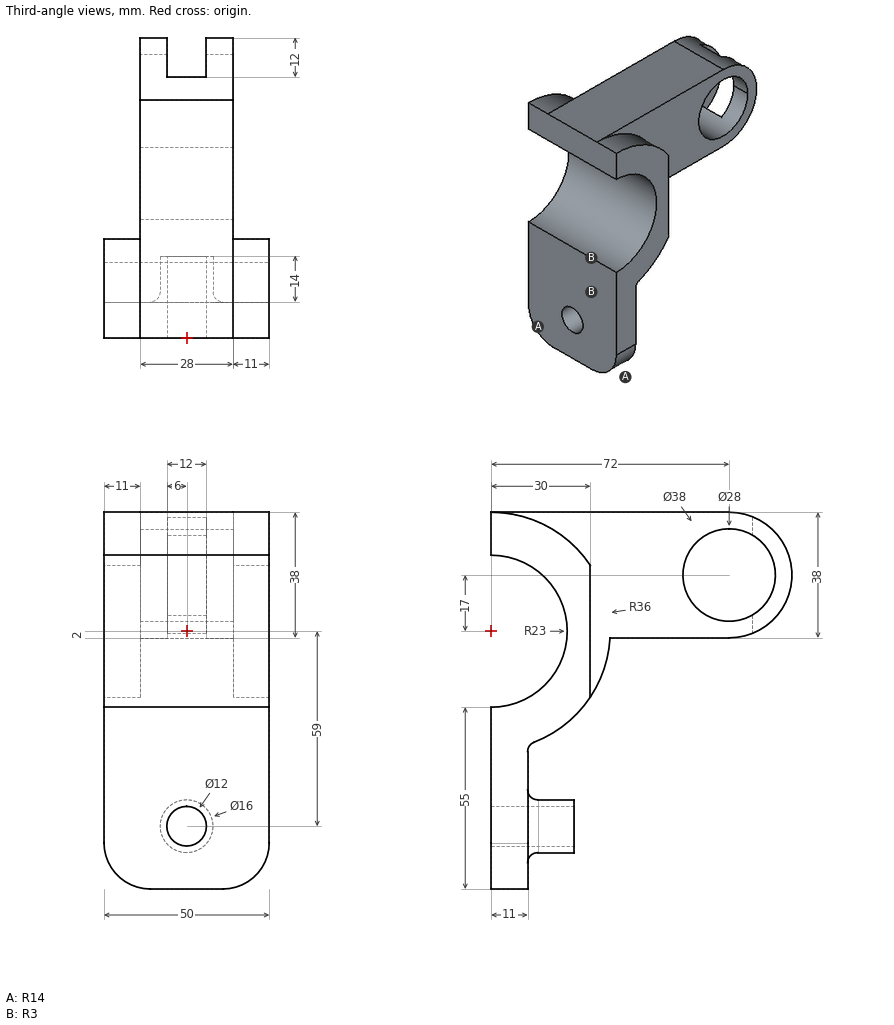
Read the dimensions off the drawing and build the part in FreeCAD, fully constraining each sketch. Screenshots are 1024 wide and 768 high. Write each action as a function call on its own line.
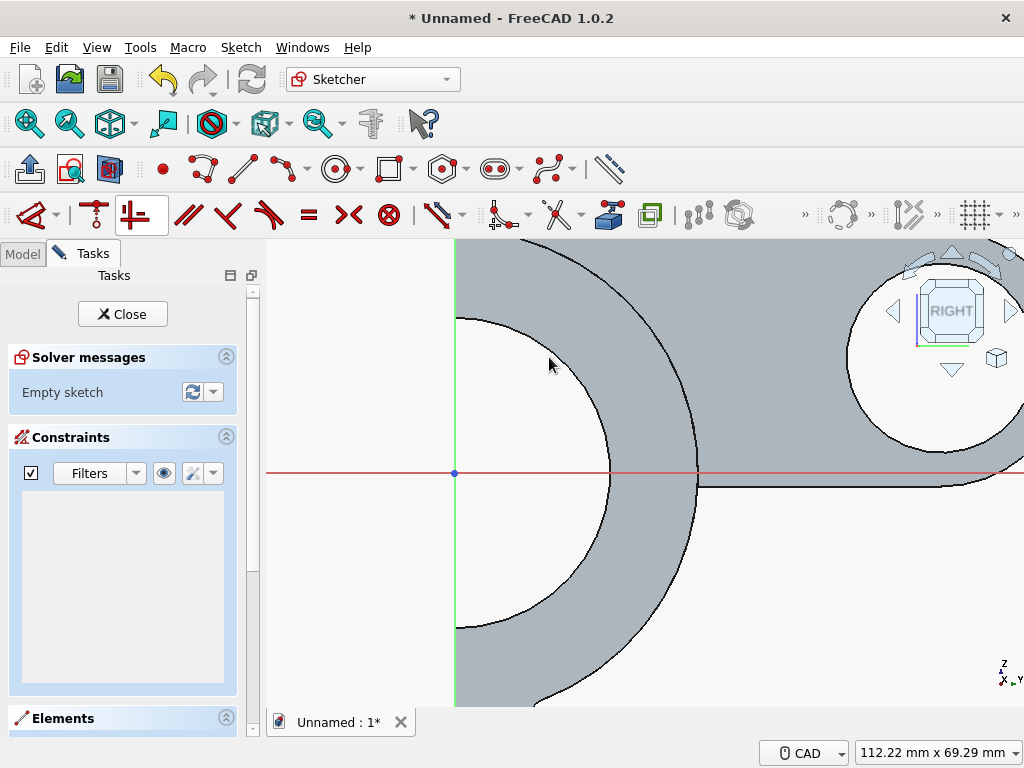
click(244, 170)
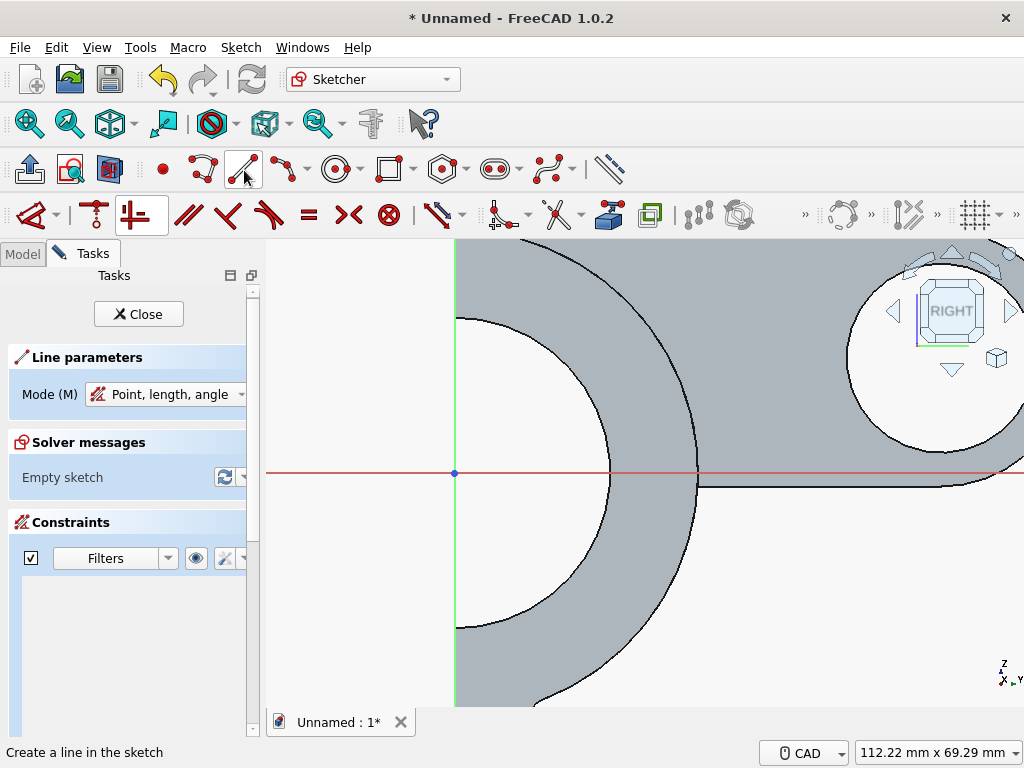
click(657, 339)
click(657, 607)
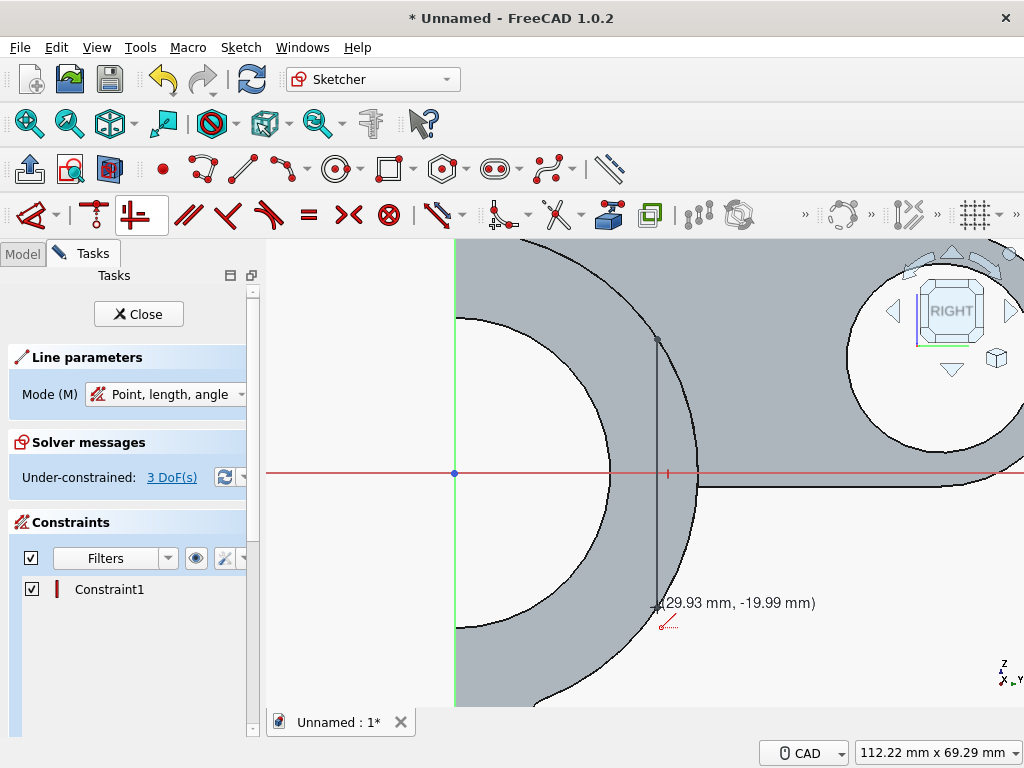
click(284, 170)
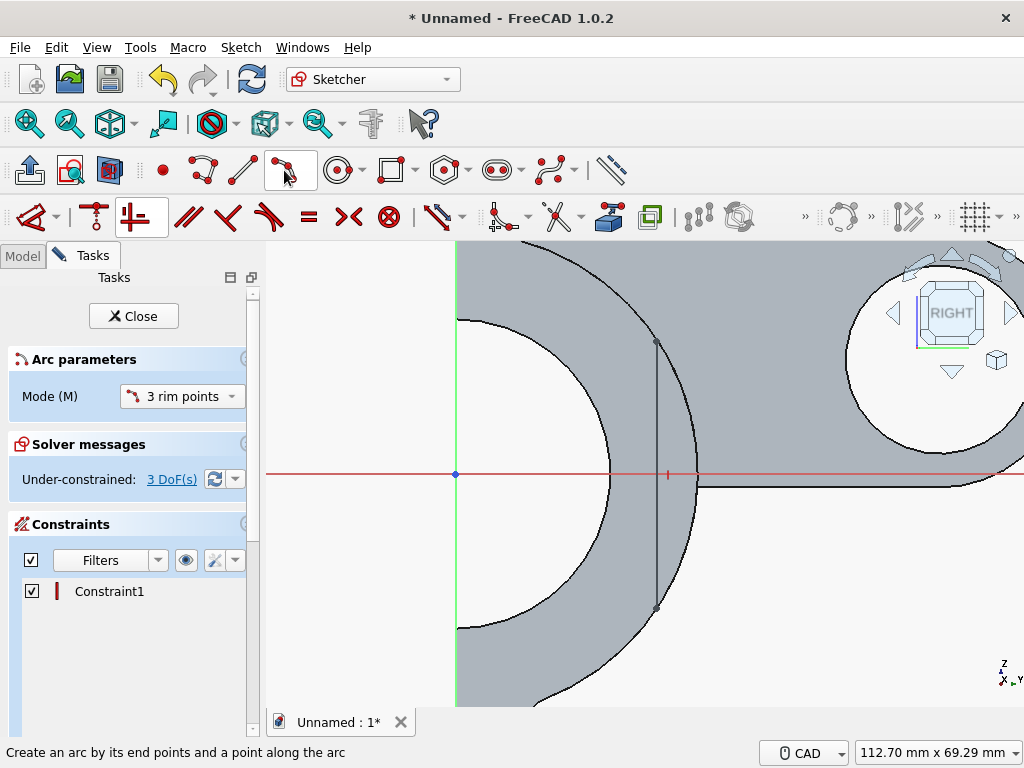
click(657, 608)
click(657, 342)
click(696, 502)
key(Escape)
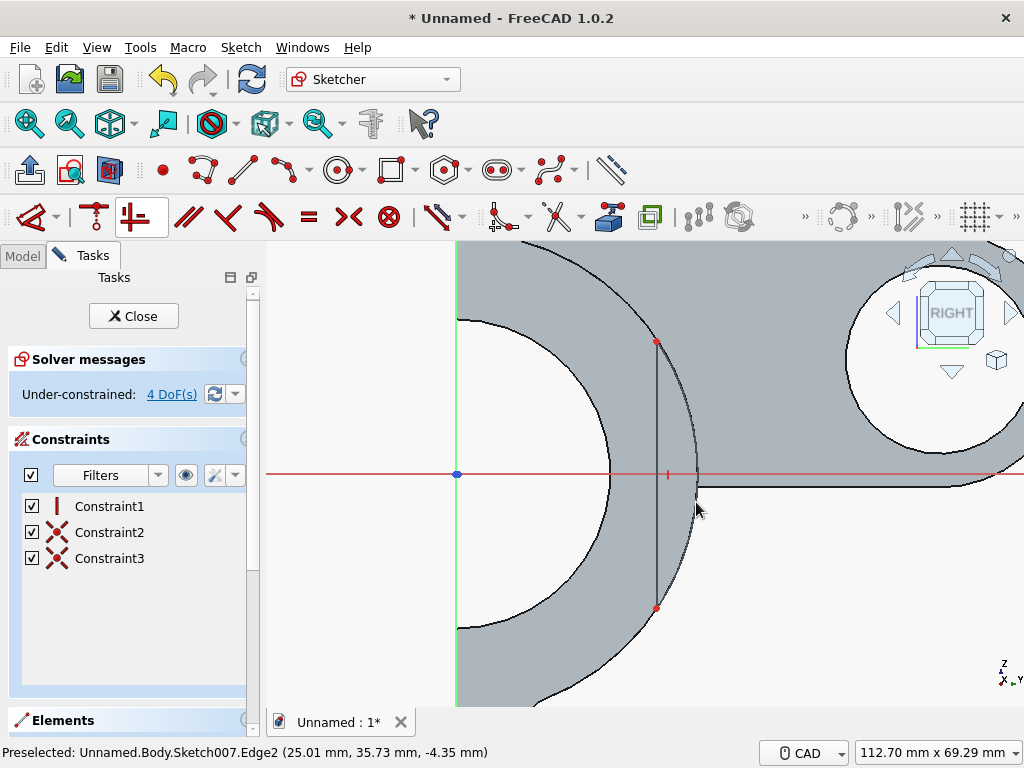
drag(446, 464, 469, 485)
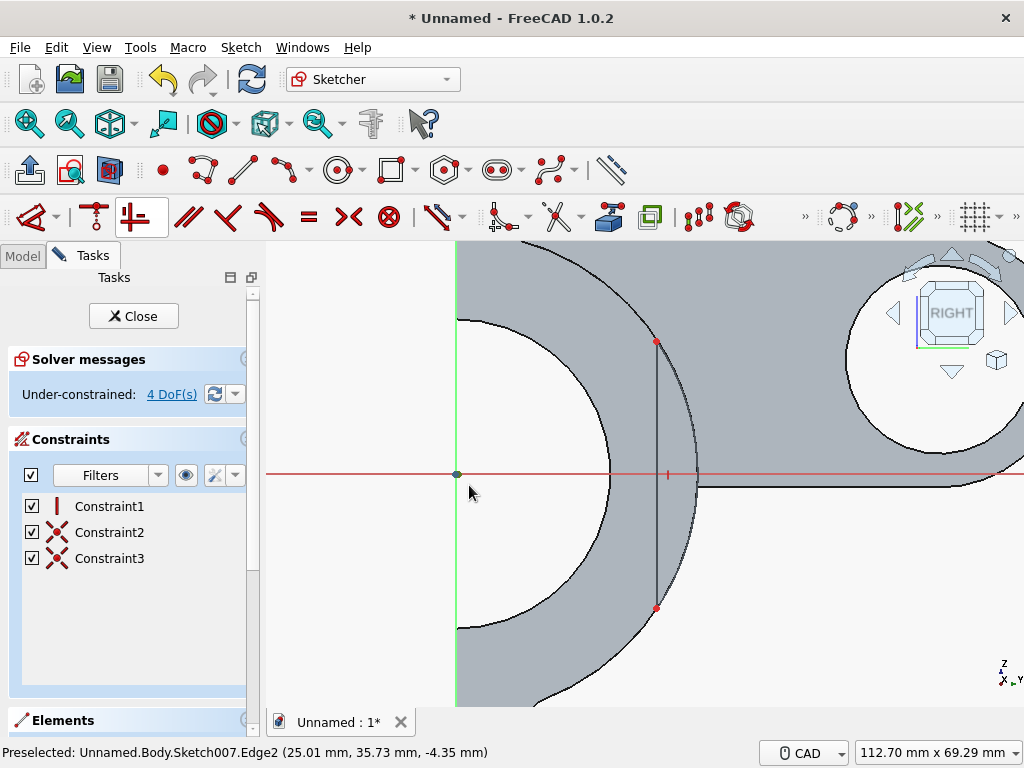
click(94, 218)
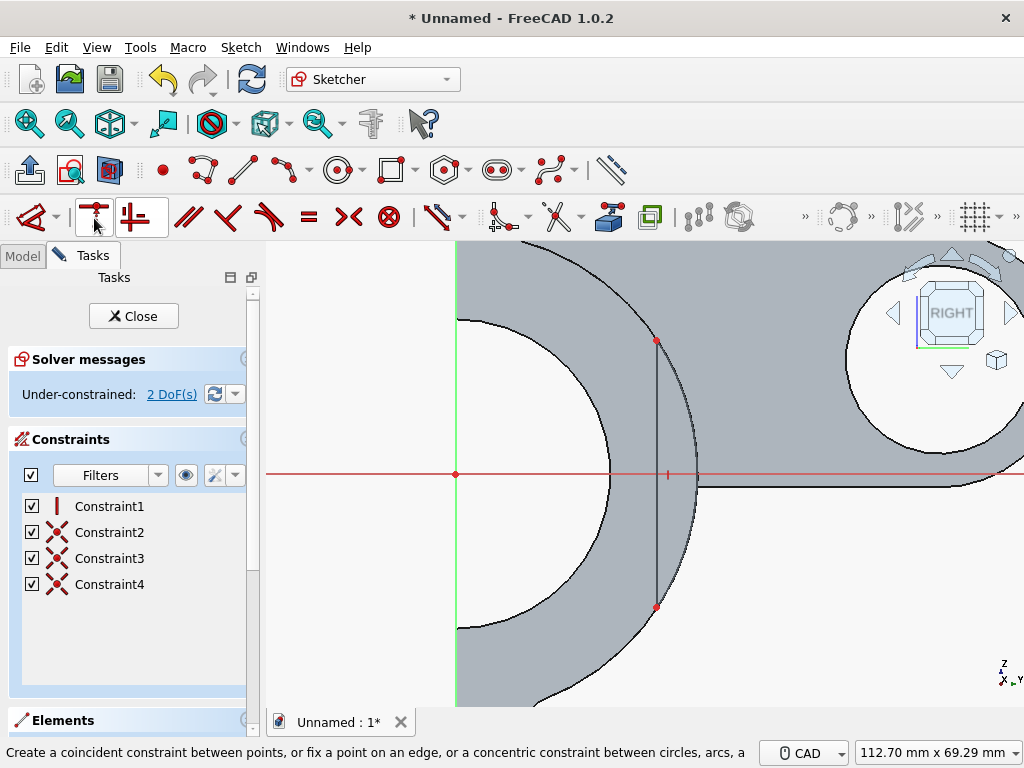
click(32, 218)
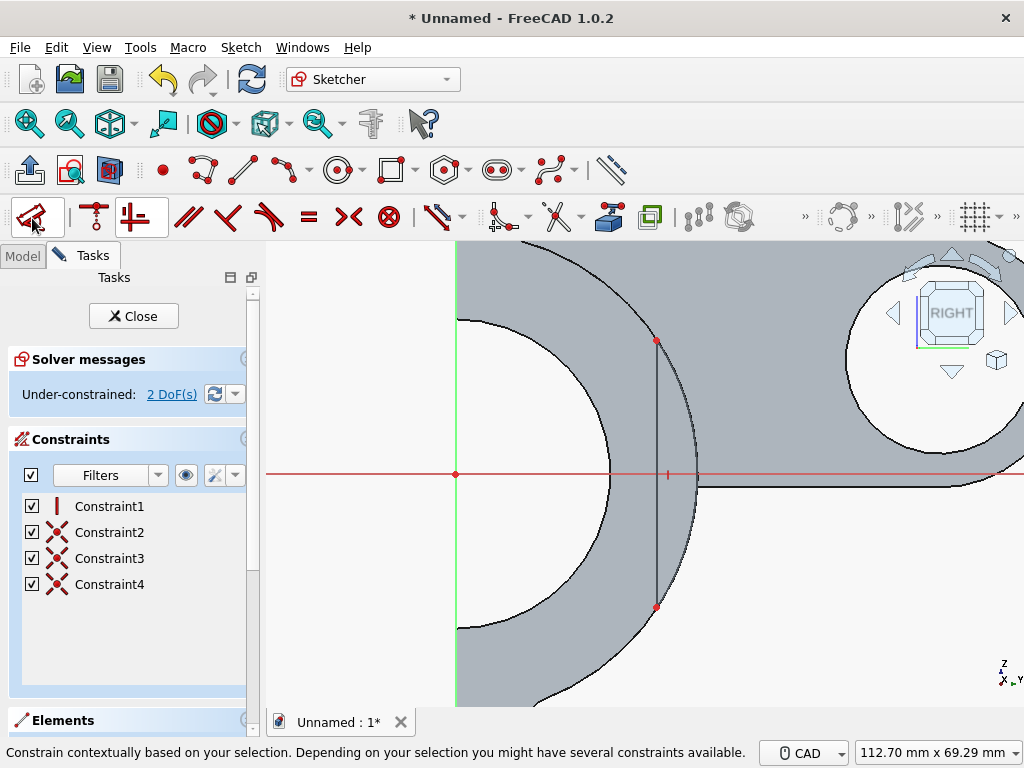
click(691, 530)
click(722, 537)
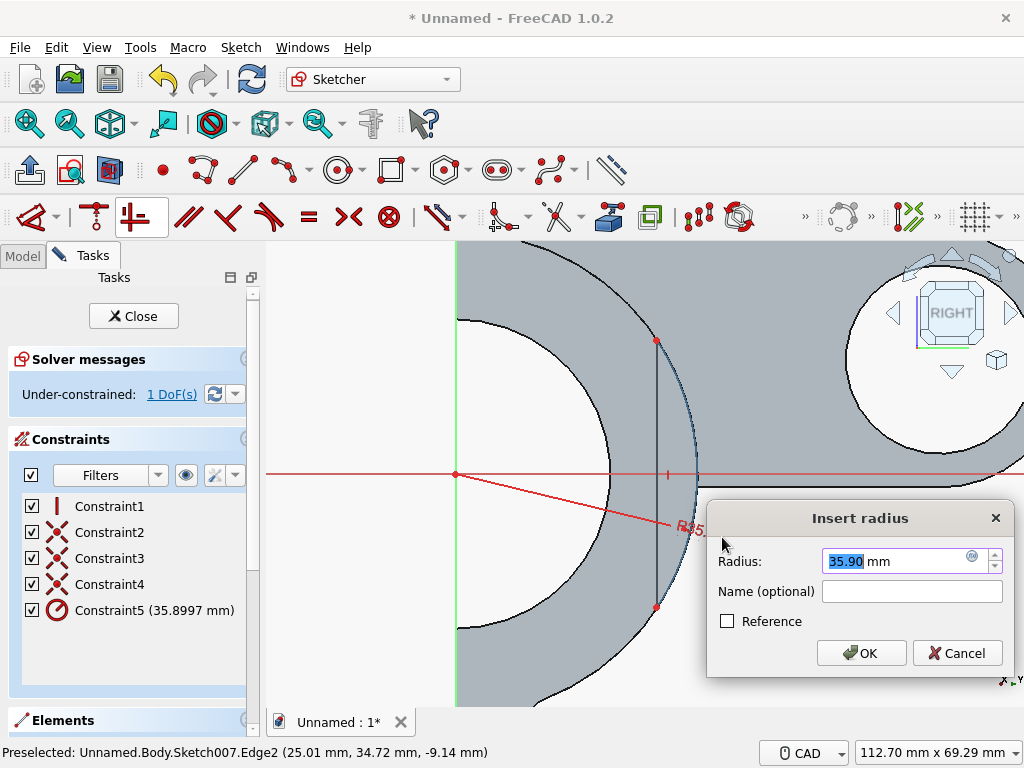
text(36)
key(Return)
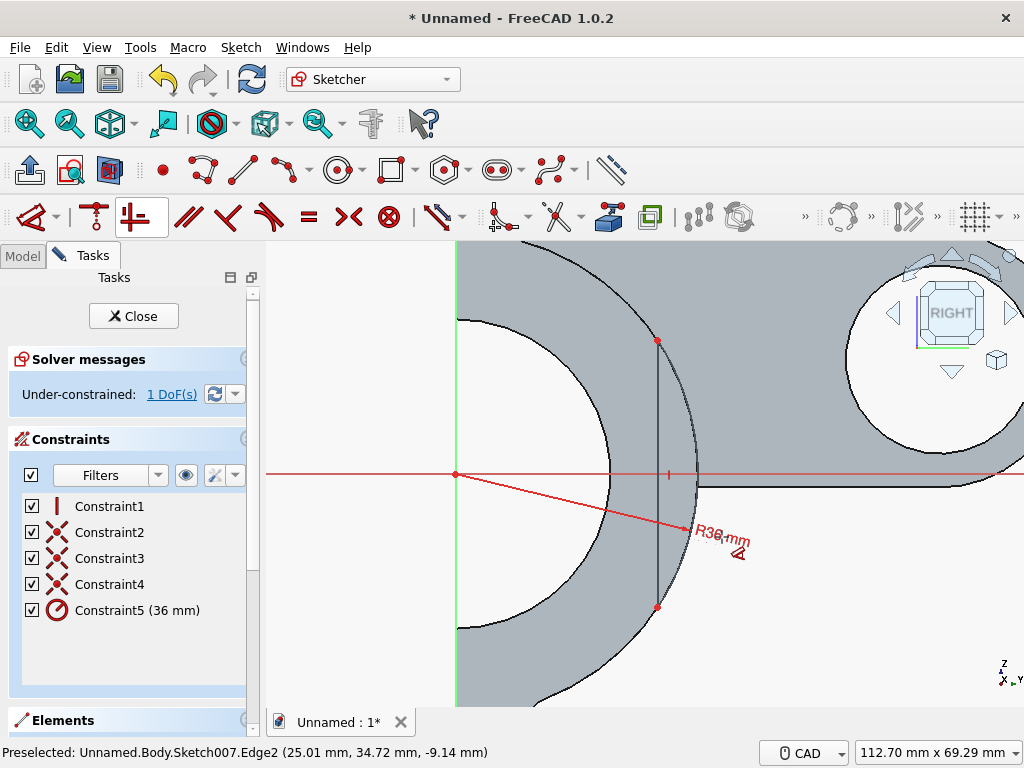
click(658, 341)
click(557, 307)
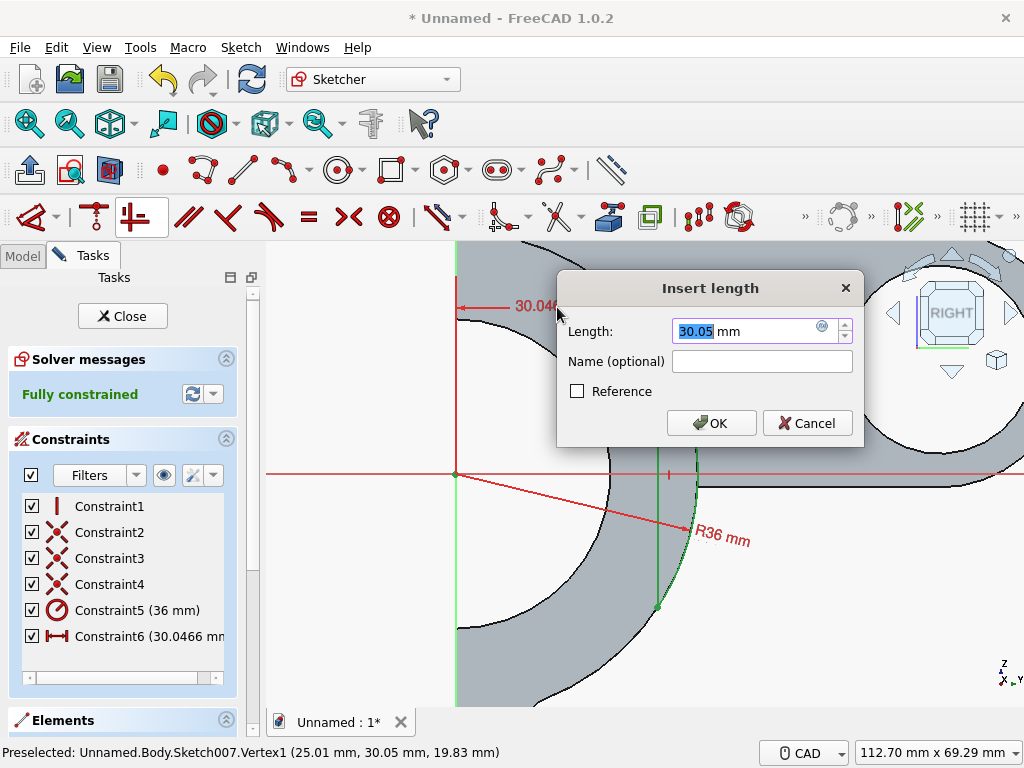
text(30)
key(Return)
key(Escape)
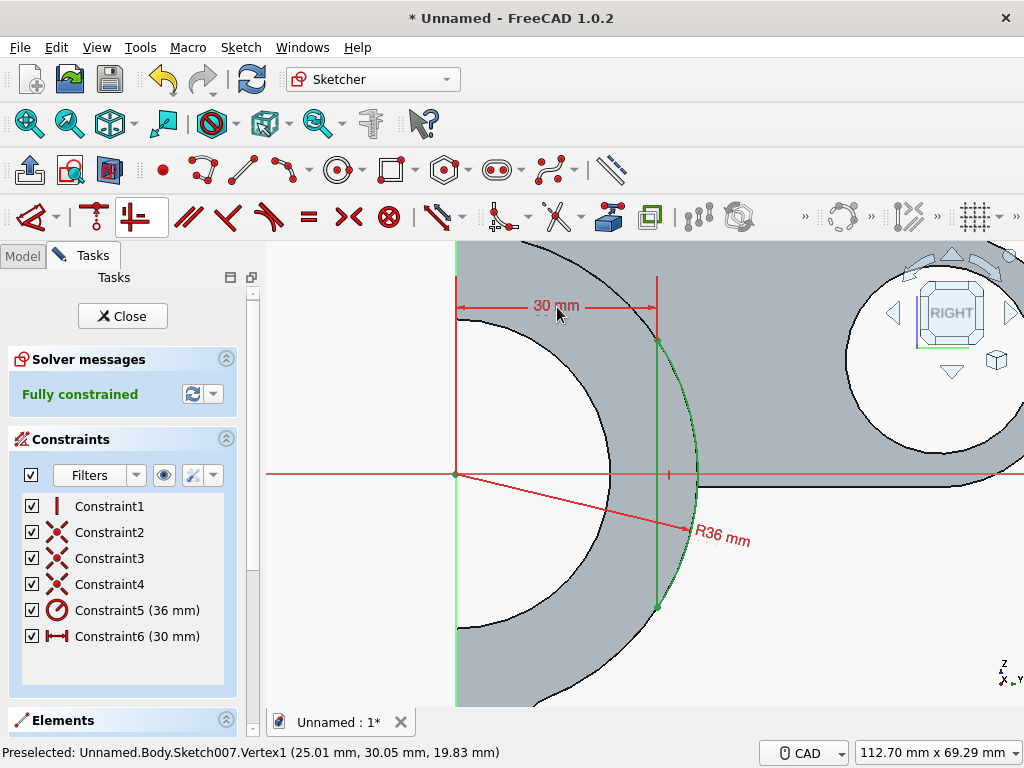
click(123, 316)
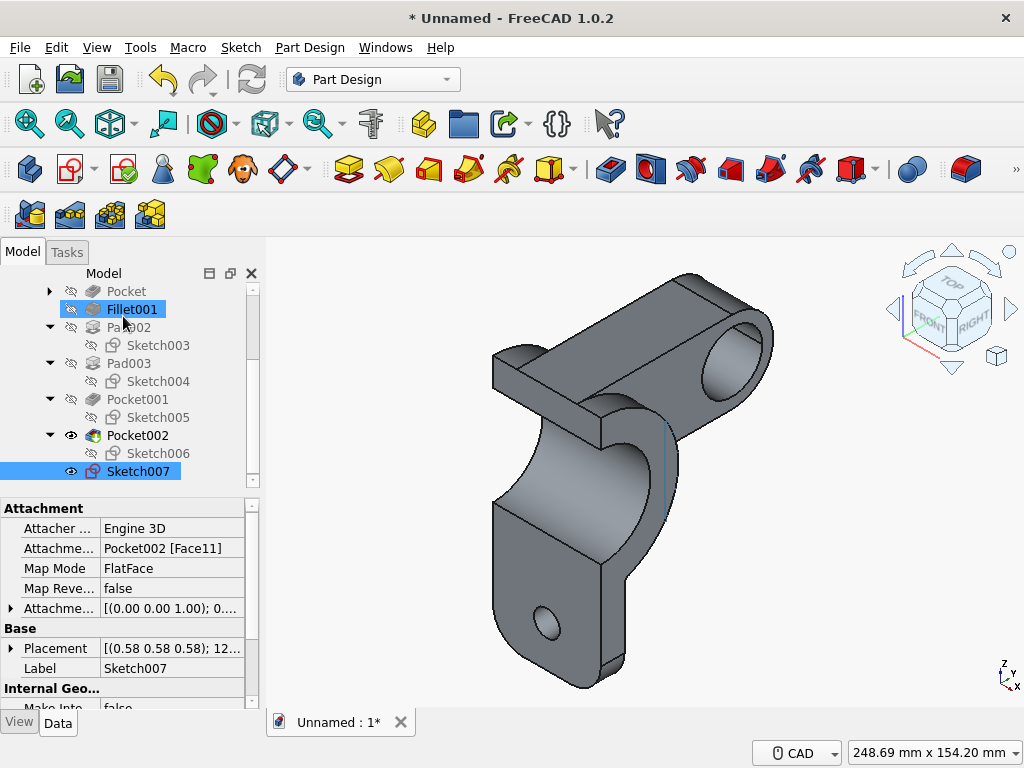
click(612, 170)